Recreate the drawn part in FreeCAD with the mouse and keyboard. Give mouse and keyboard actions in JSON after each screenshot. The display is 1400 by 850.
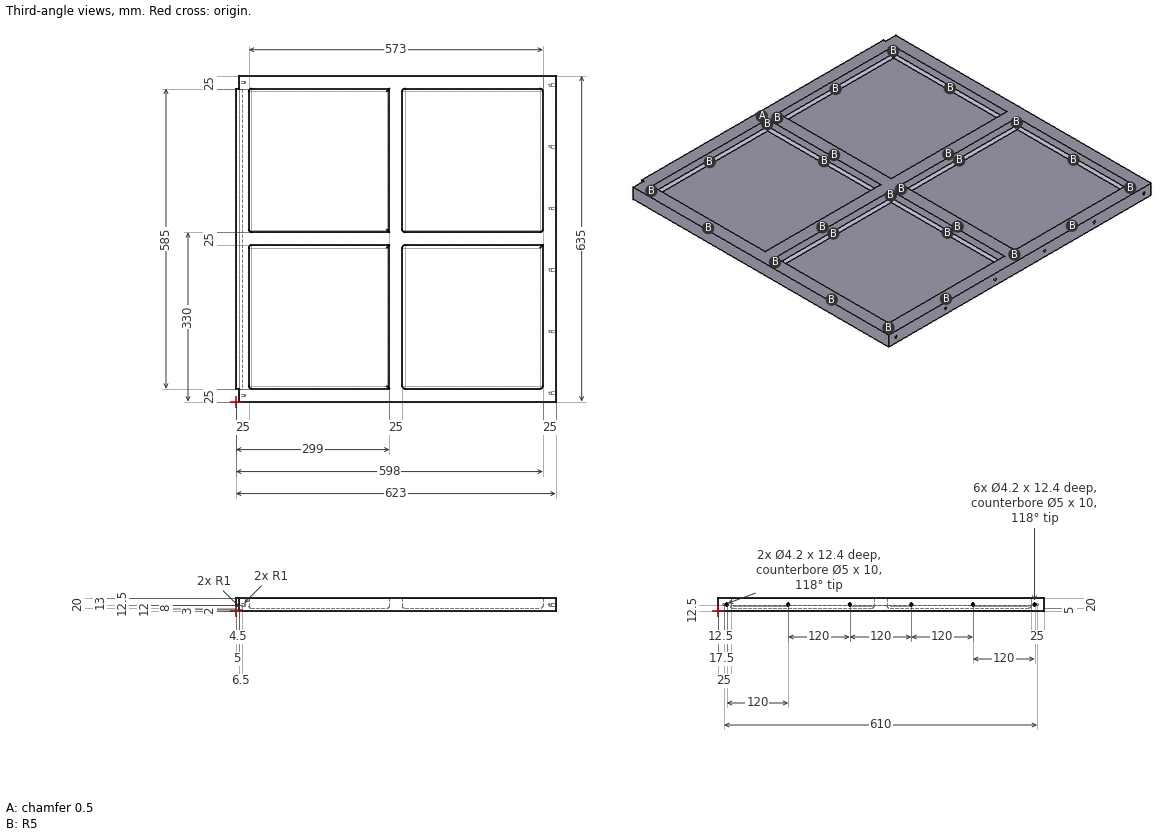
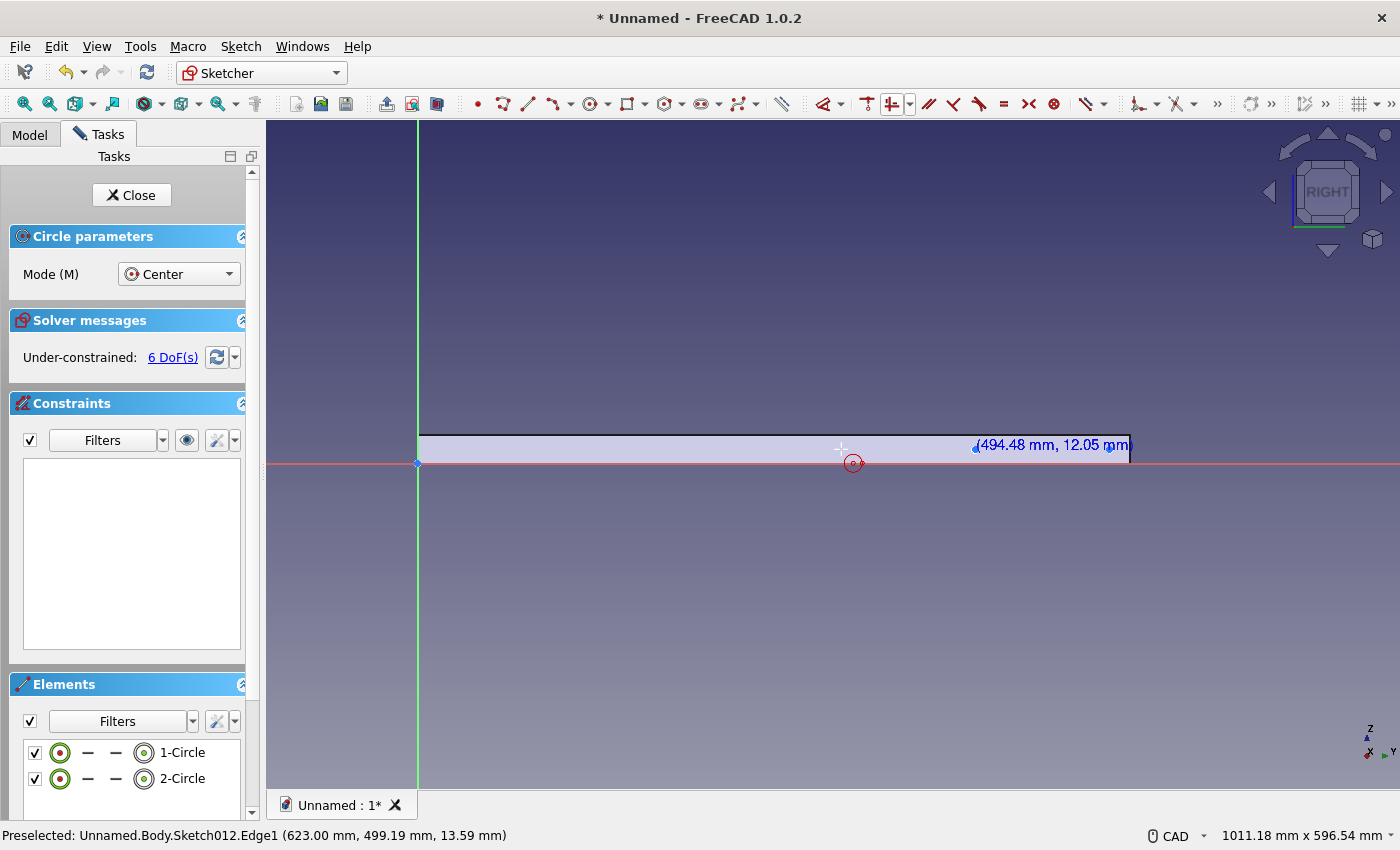
{"action": "left_click", "coordinate": [841, 449]}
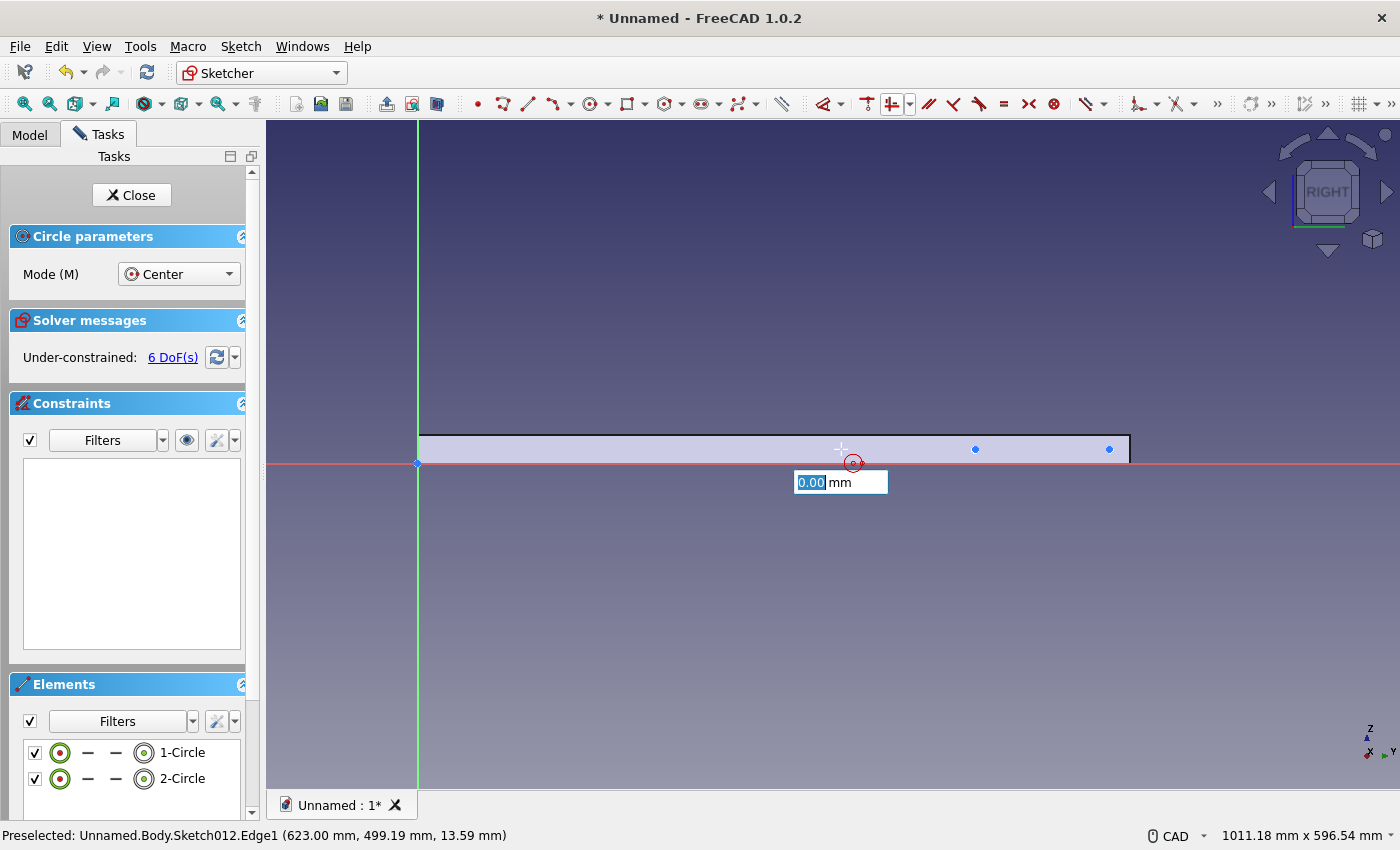
{"action": "scroll", "coordinate": [843, 448], "scroll_direction": "up", "scroll_amount": 10}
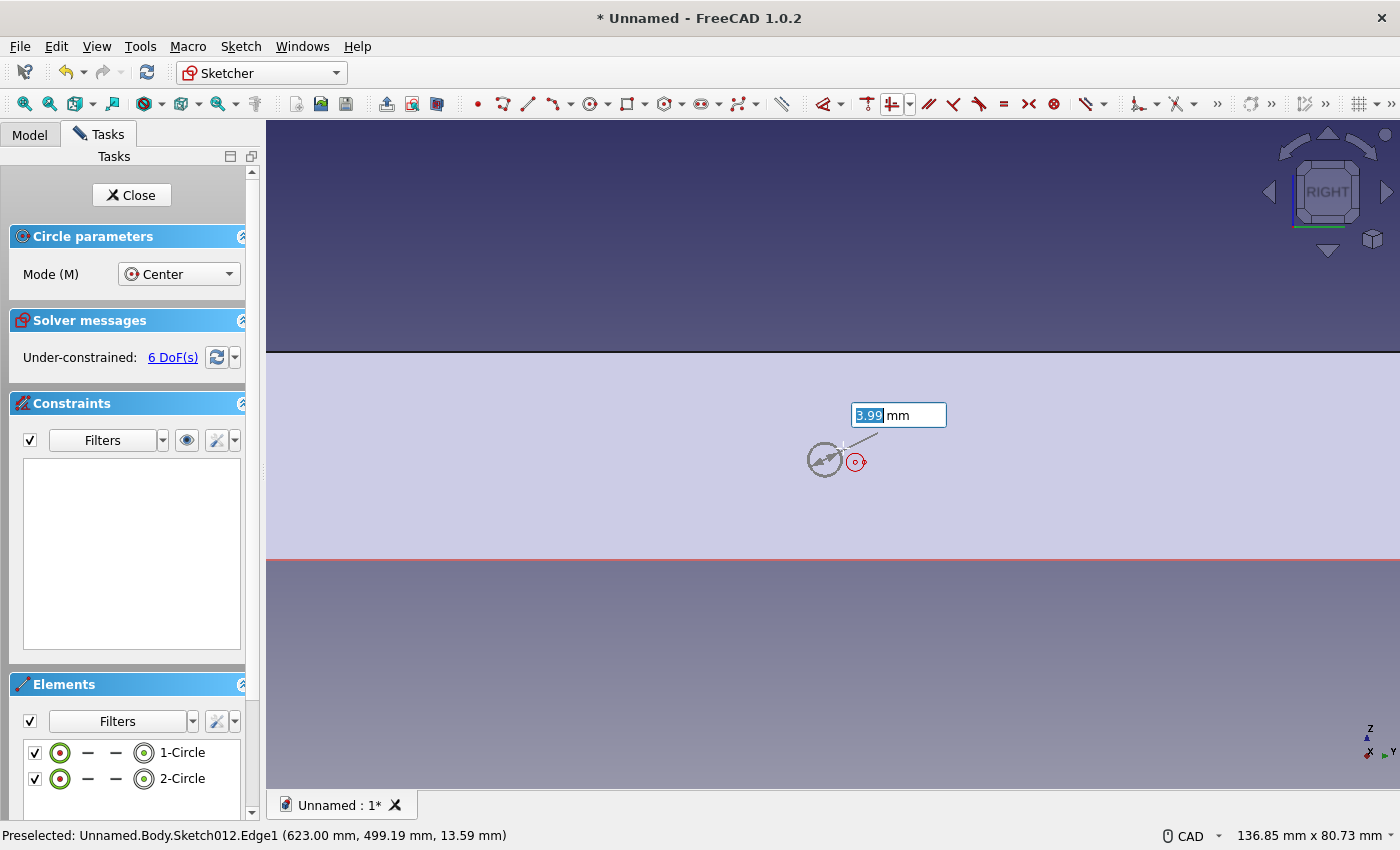
{"action": "left_click", "coordinate": [837, 444]}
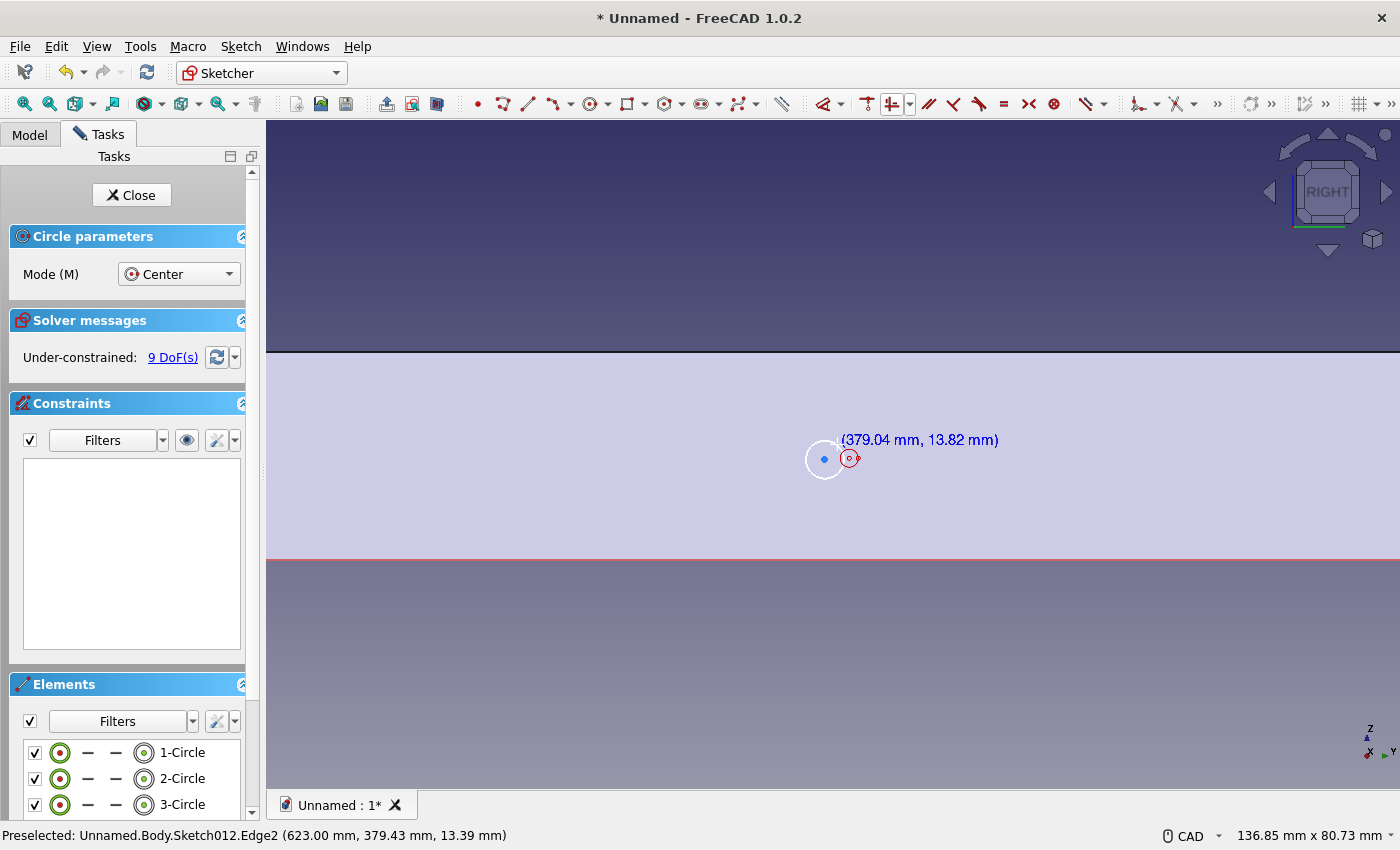
{"action": "scroll", "coordinate": [843, 448], "scroll_direction": "down", "scroll_amount": 10}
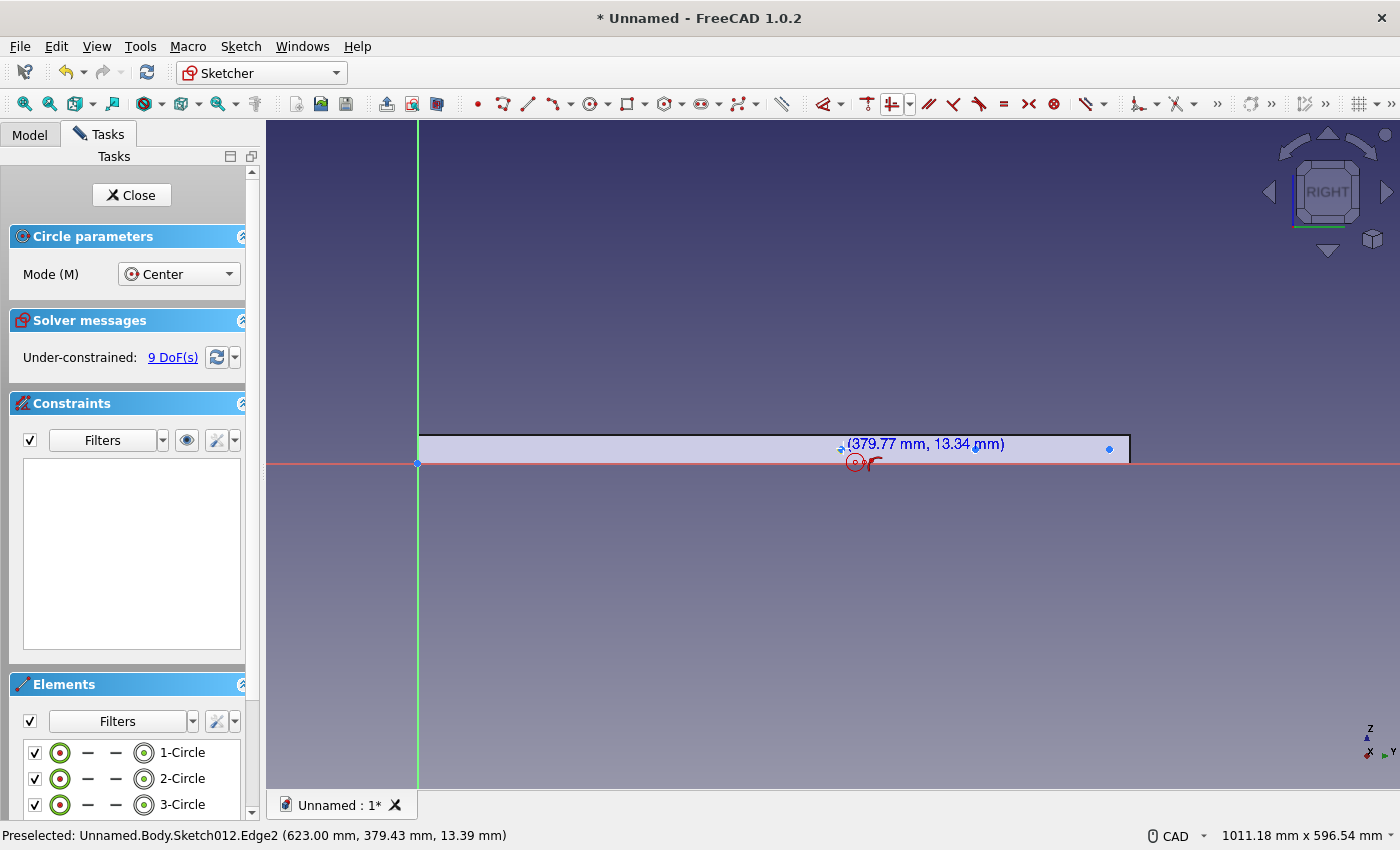
{"action": "scroll", "coordinate": [706, 449], "scroll_direction": "up", "scroll_amount": 12}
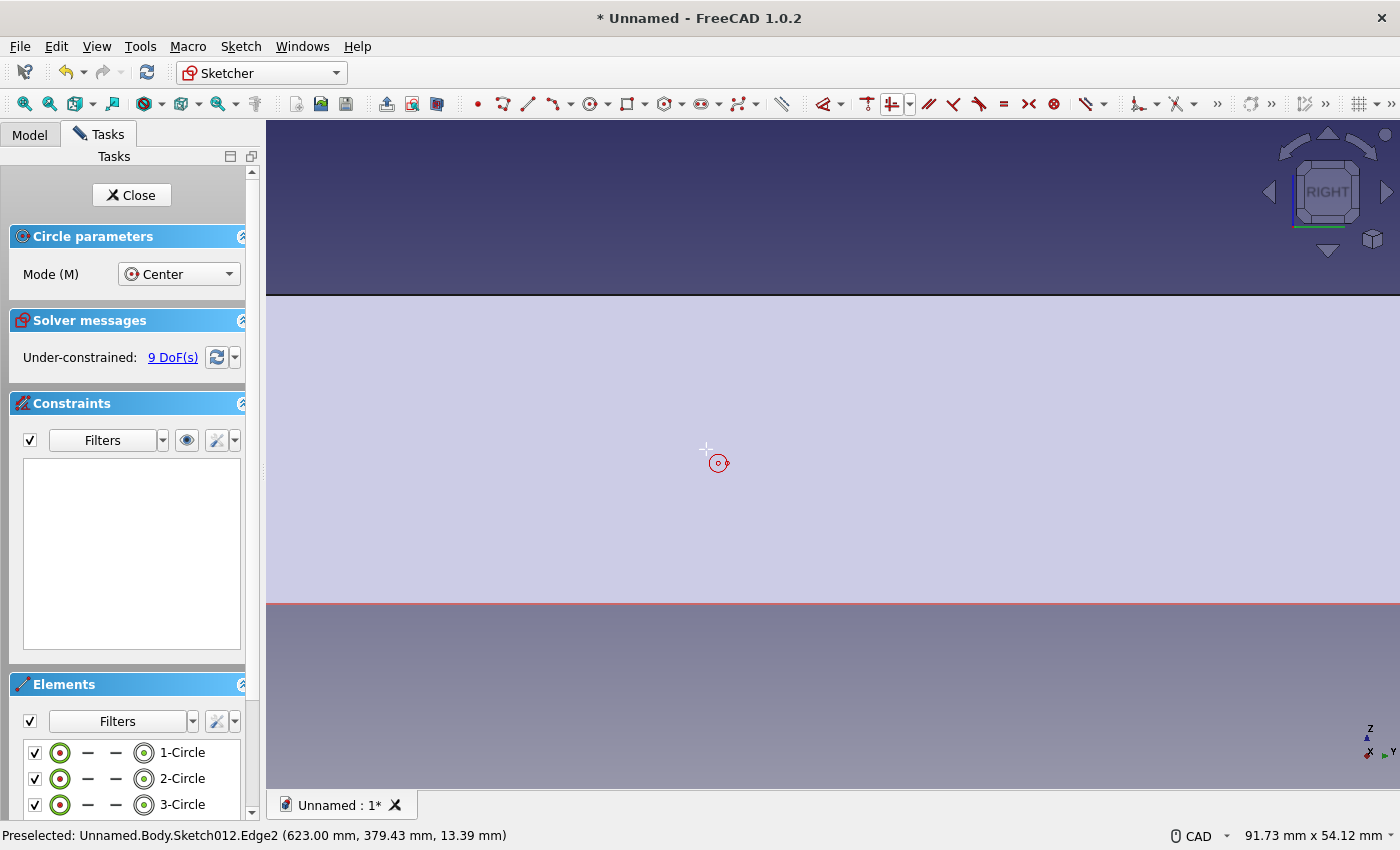
{"action": "scroll", "coordinate": [706, 449], "scroll_direction": "down", "scroll_amount": 12}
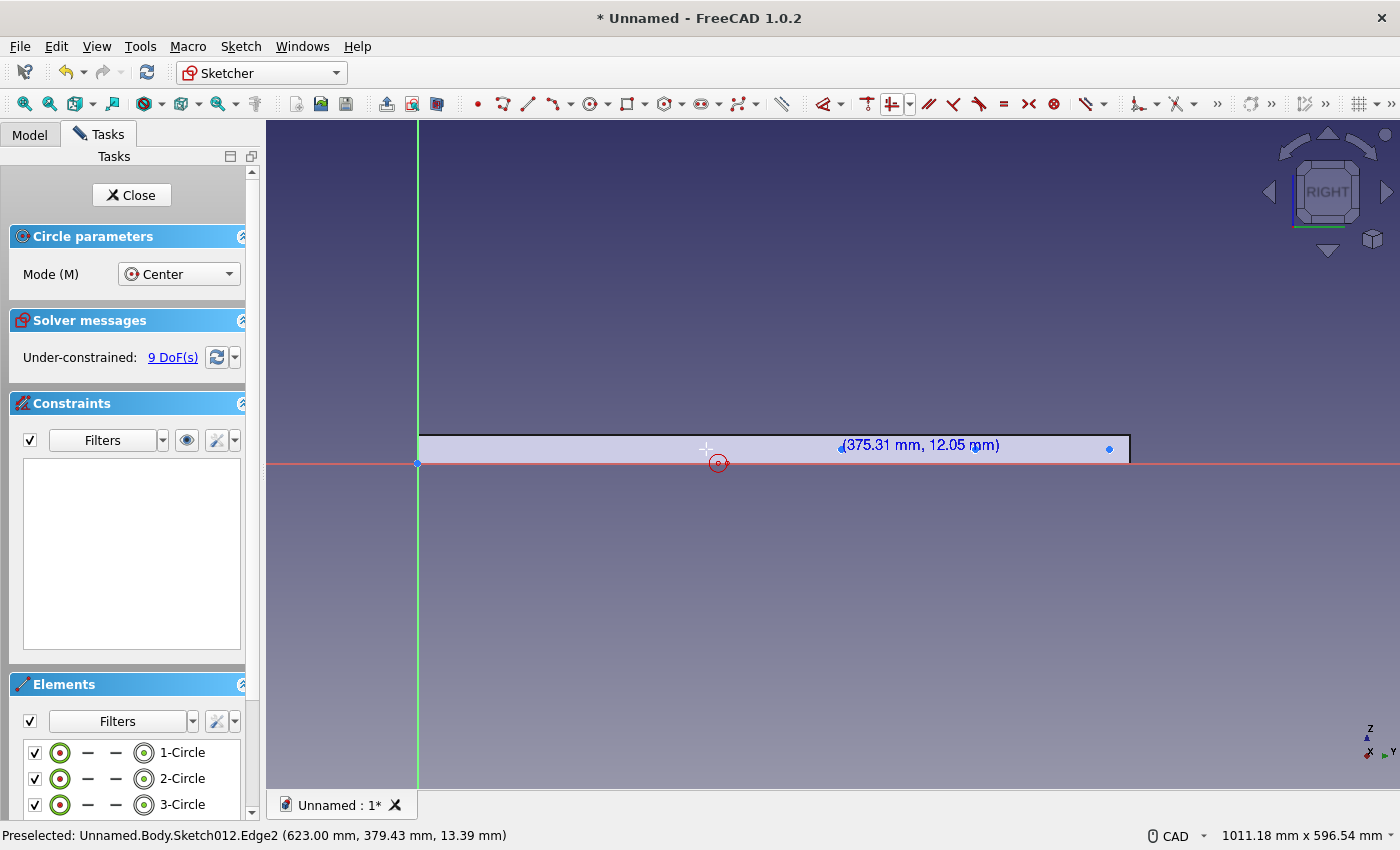
{"action": "left_click", "coordinate": [706, 449]}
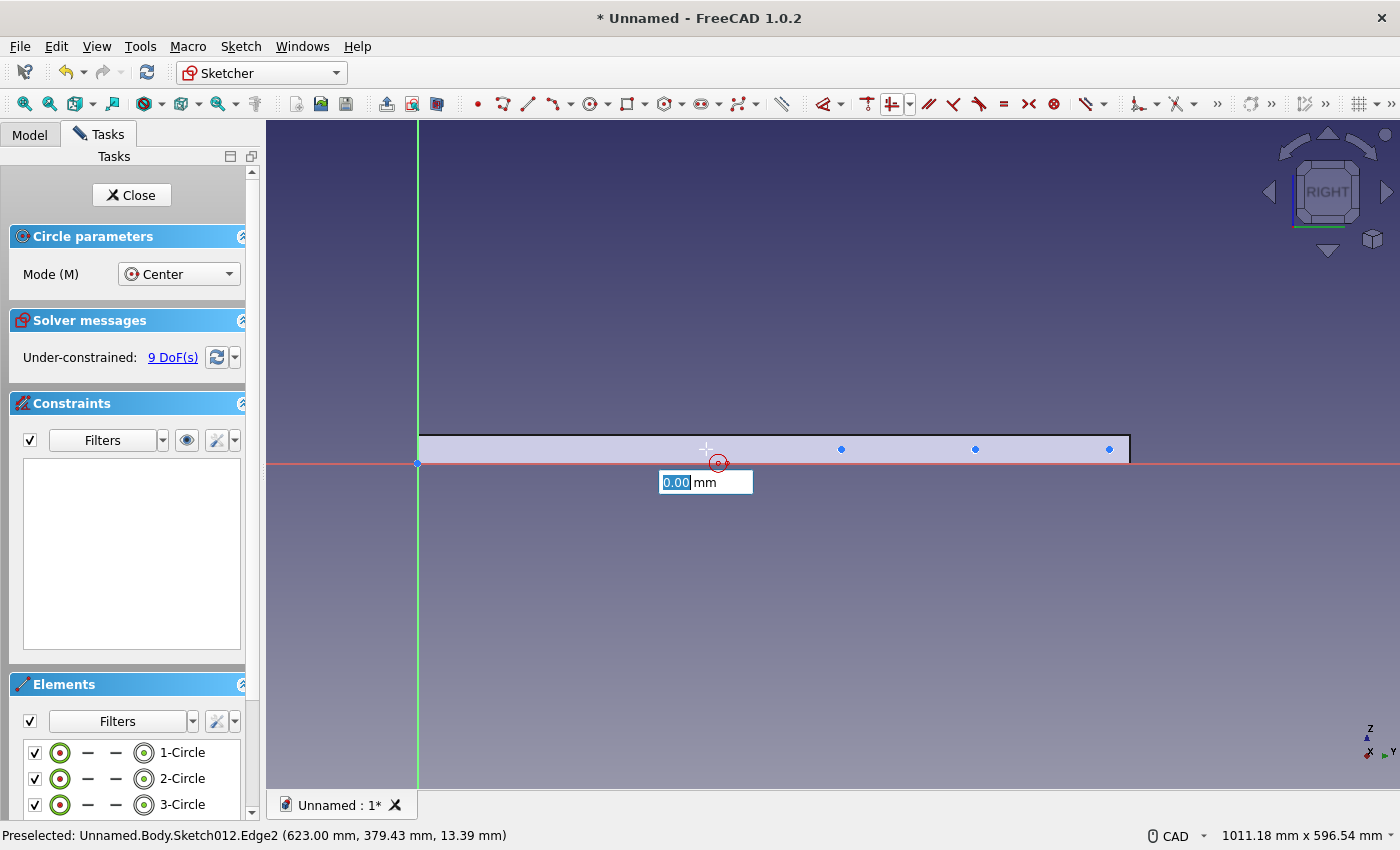
{"action": "scroll", "coordinate": [708, 448], "scroll_direction": "up", "scroll_amount": 10}